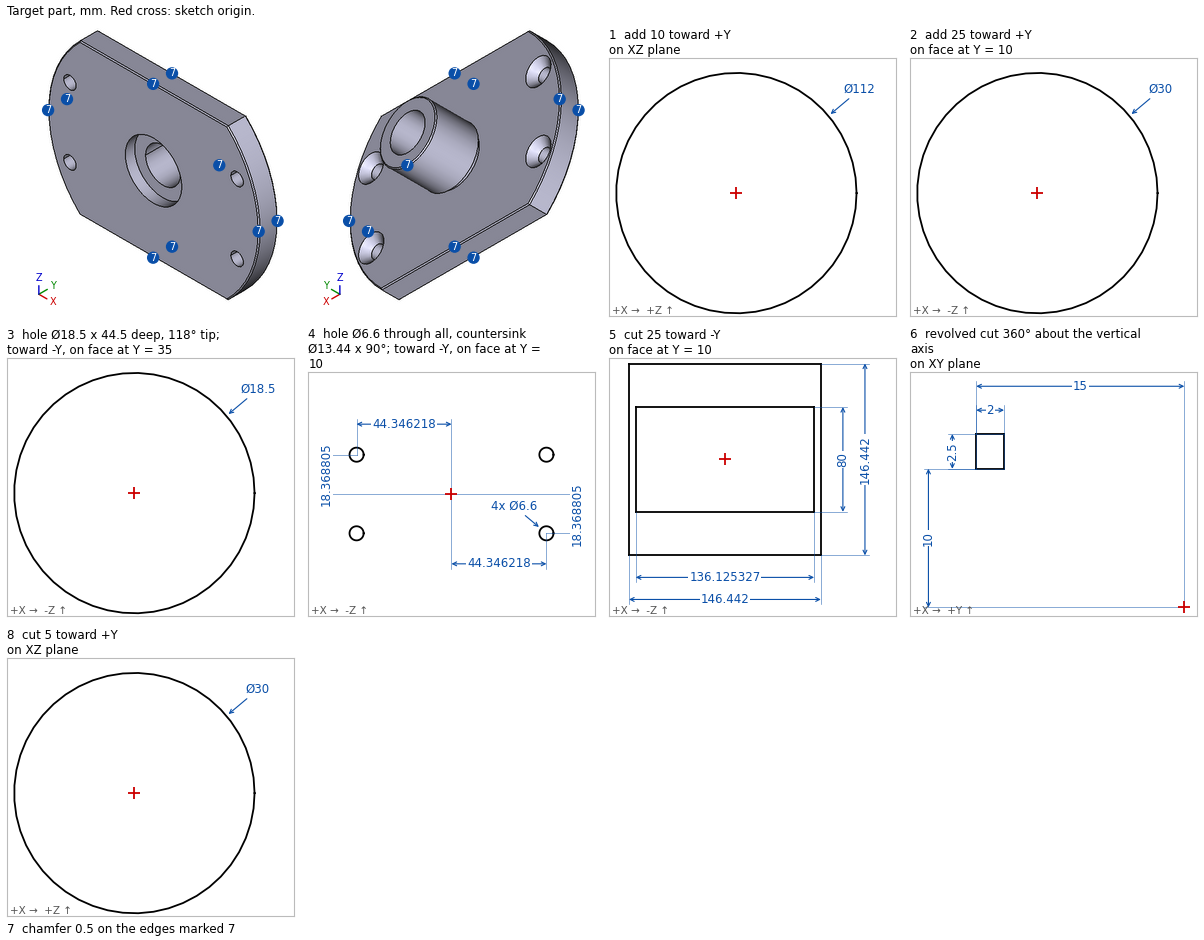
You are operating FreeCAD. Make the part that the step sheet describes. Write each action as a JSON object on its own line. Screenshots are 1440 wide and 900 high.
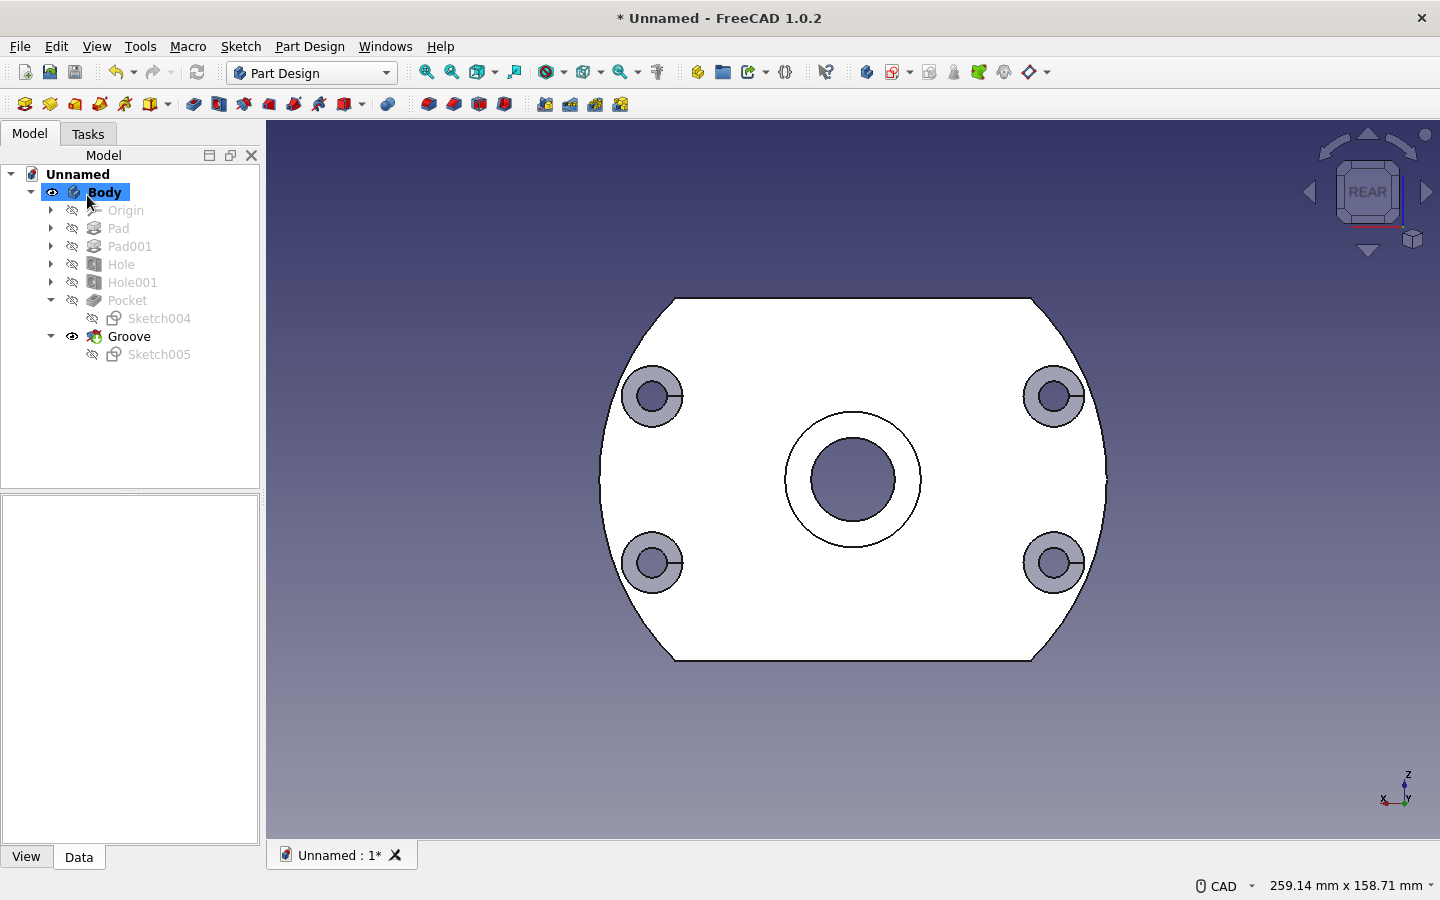
{"action": "left_click", "coordinate": [638, 613]}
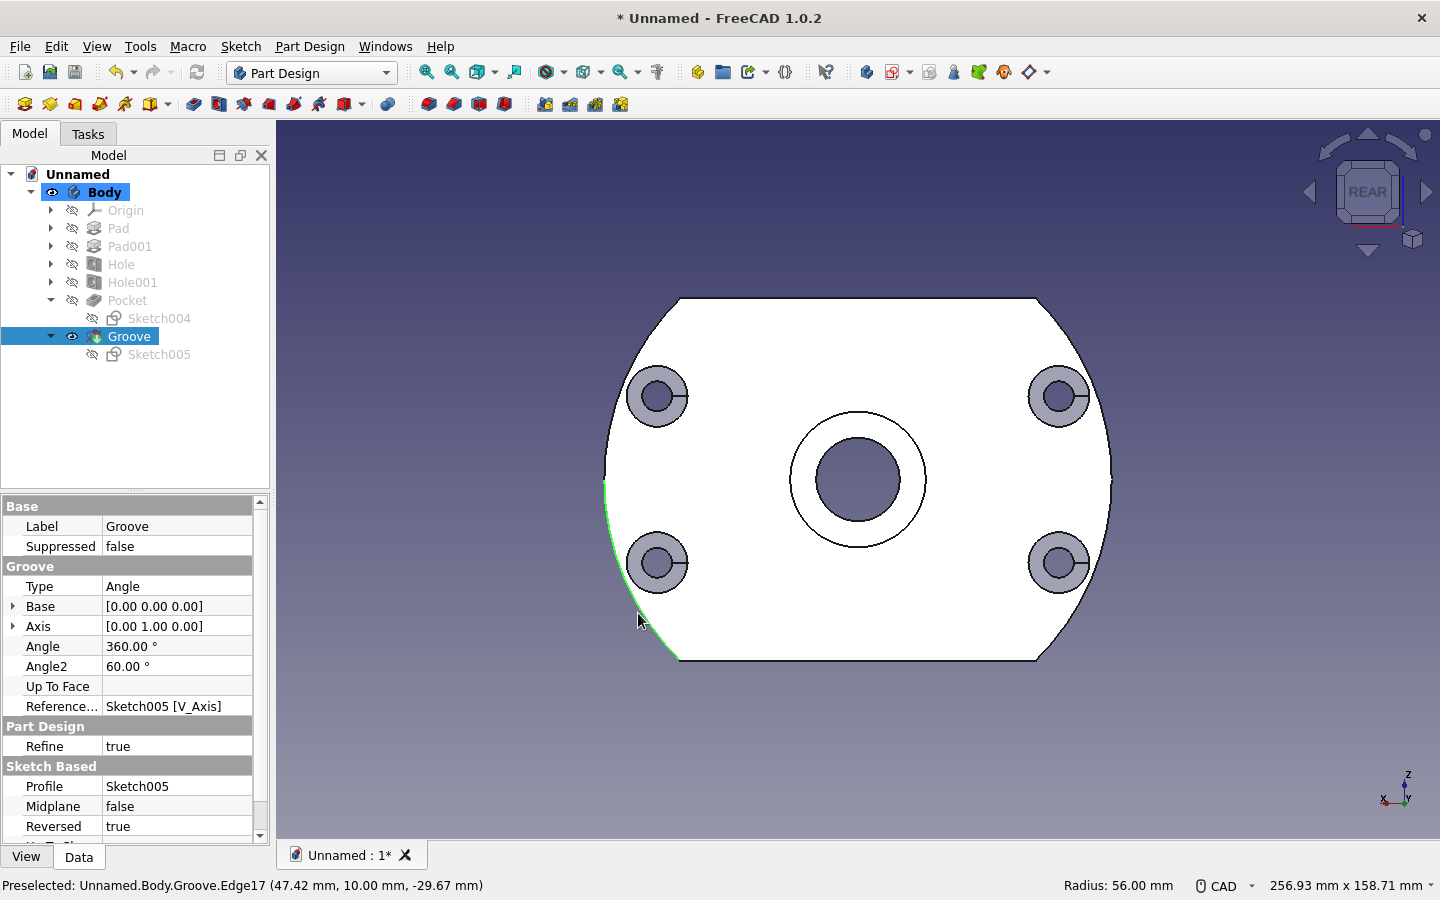
{"action": "left_click", "coordinate": [1112, 479], "text": "ctrl"}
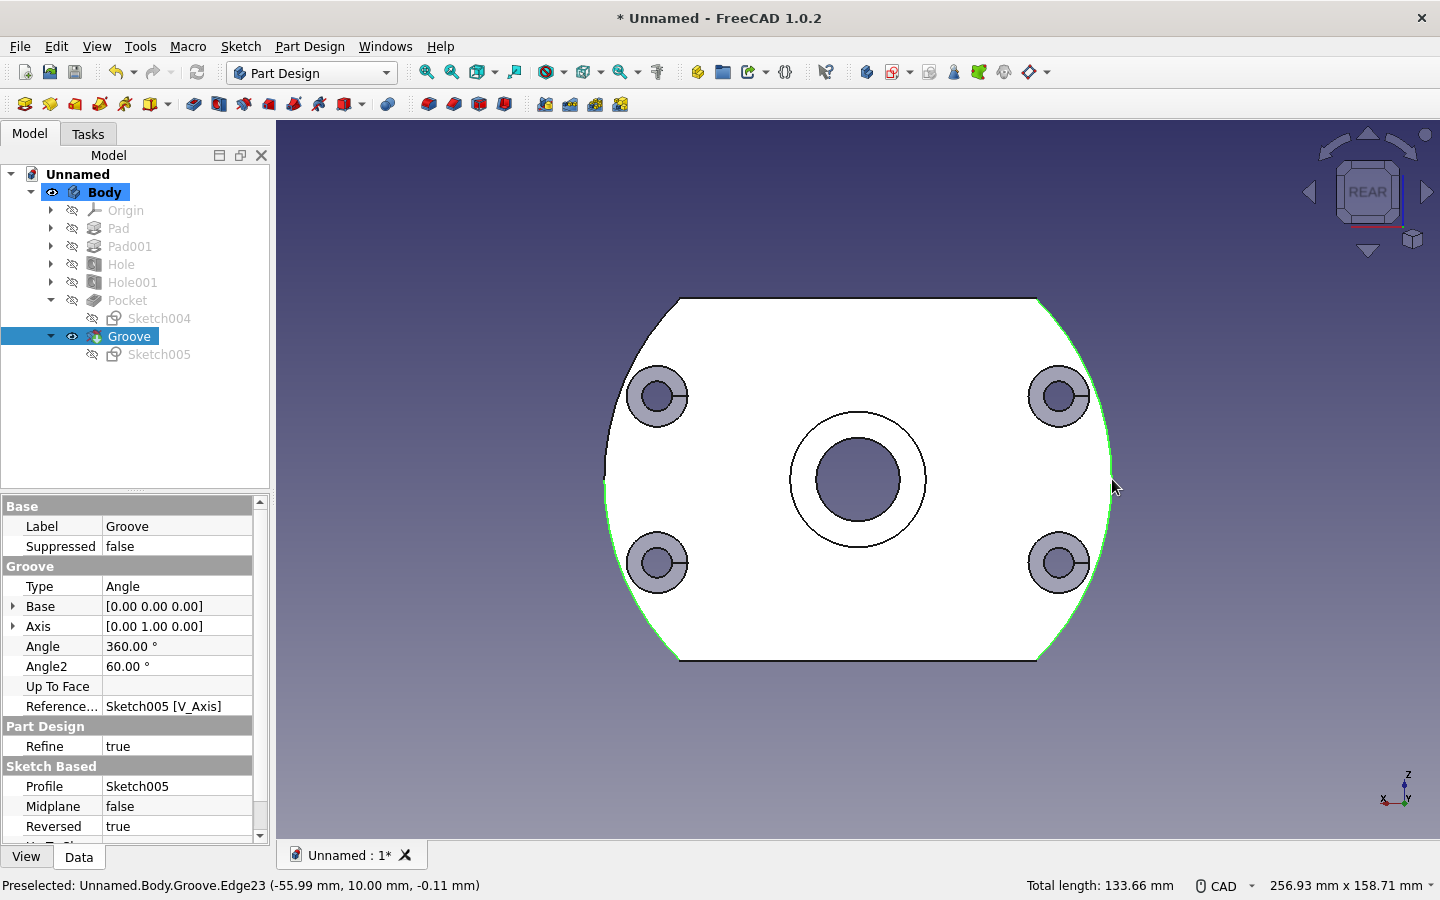
{"action": "left_click", "coordinate": [858, 660], "text": "ctrl"}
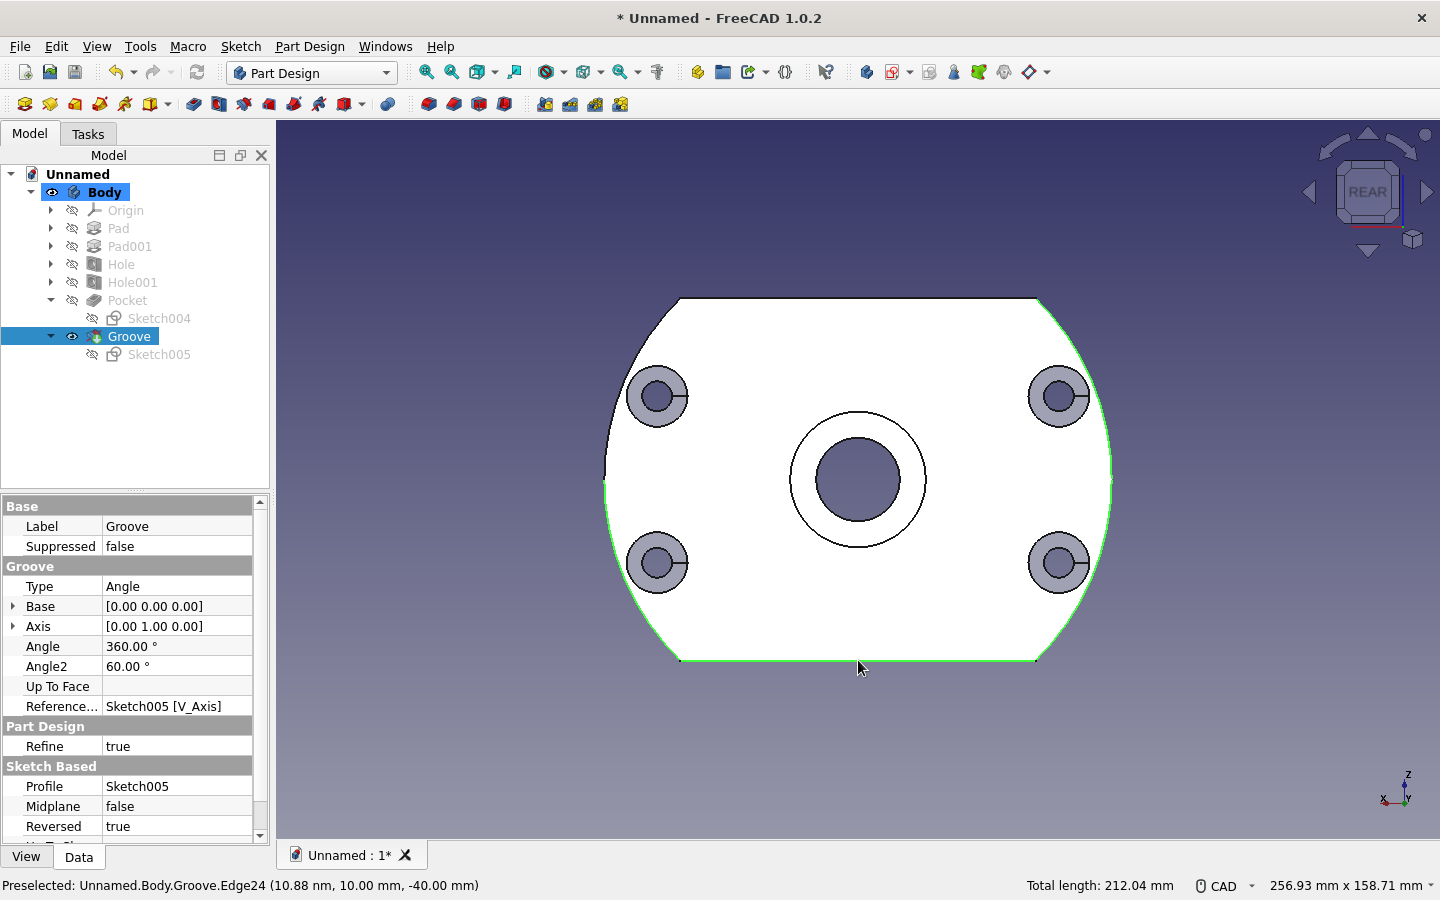
{"action": "left_click", "coordinate": [926, 478], "text": "ctrl"}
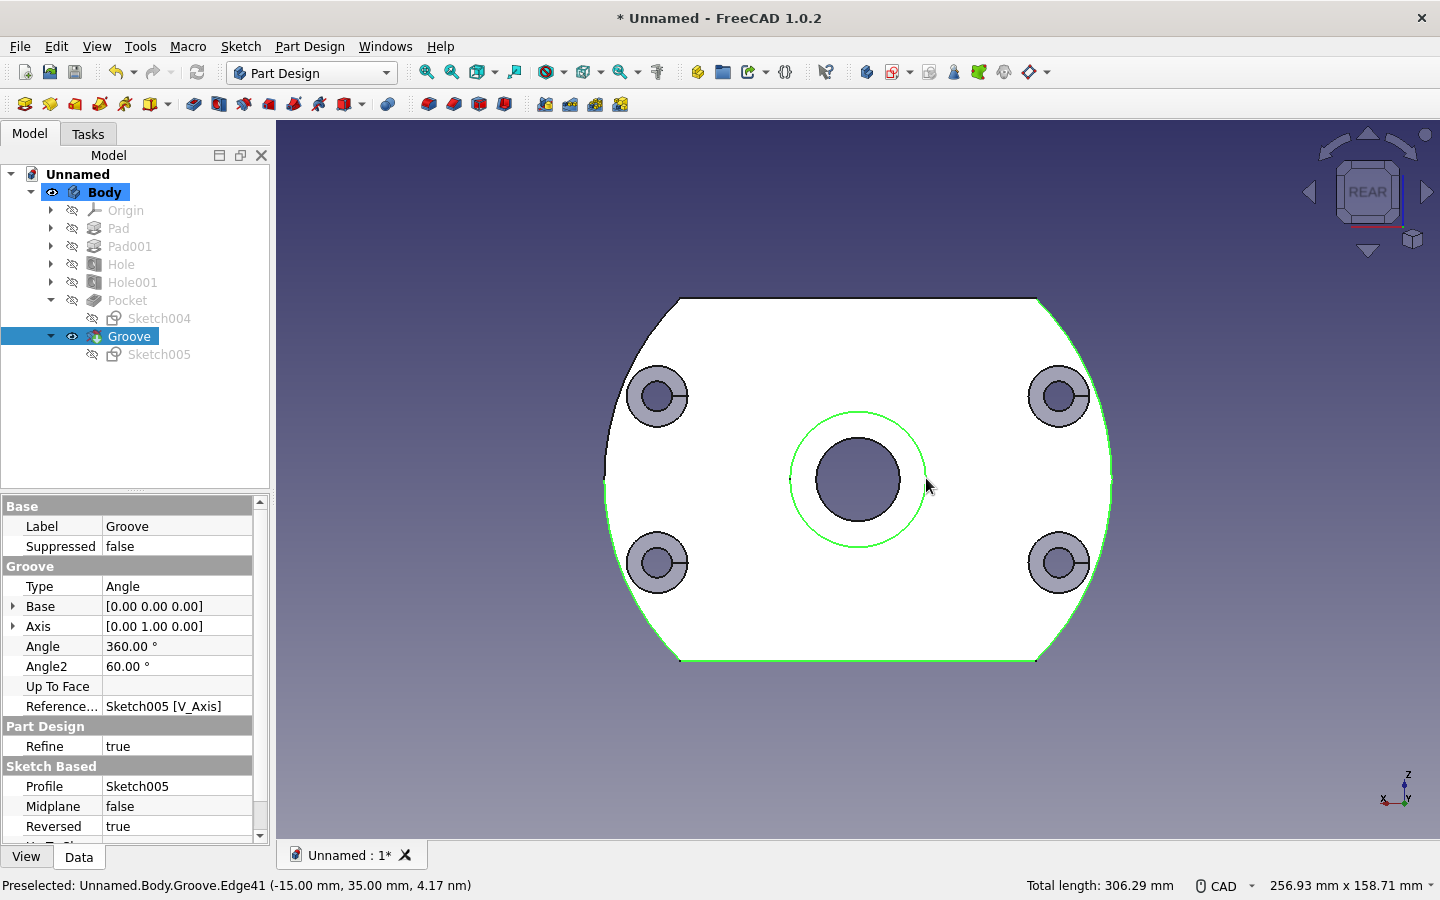
{"action": "key", "text": "0"}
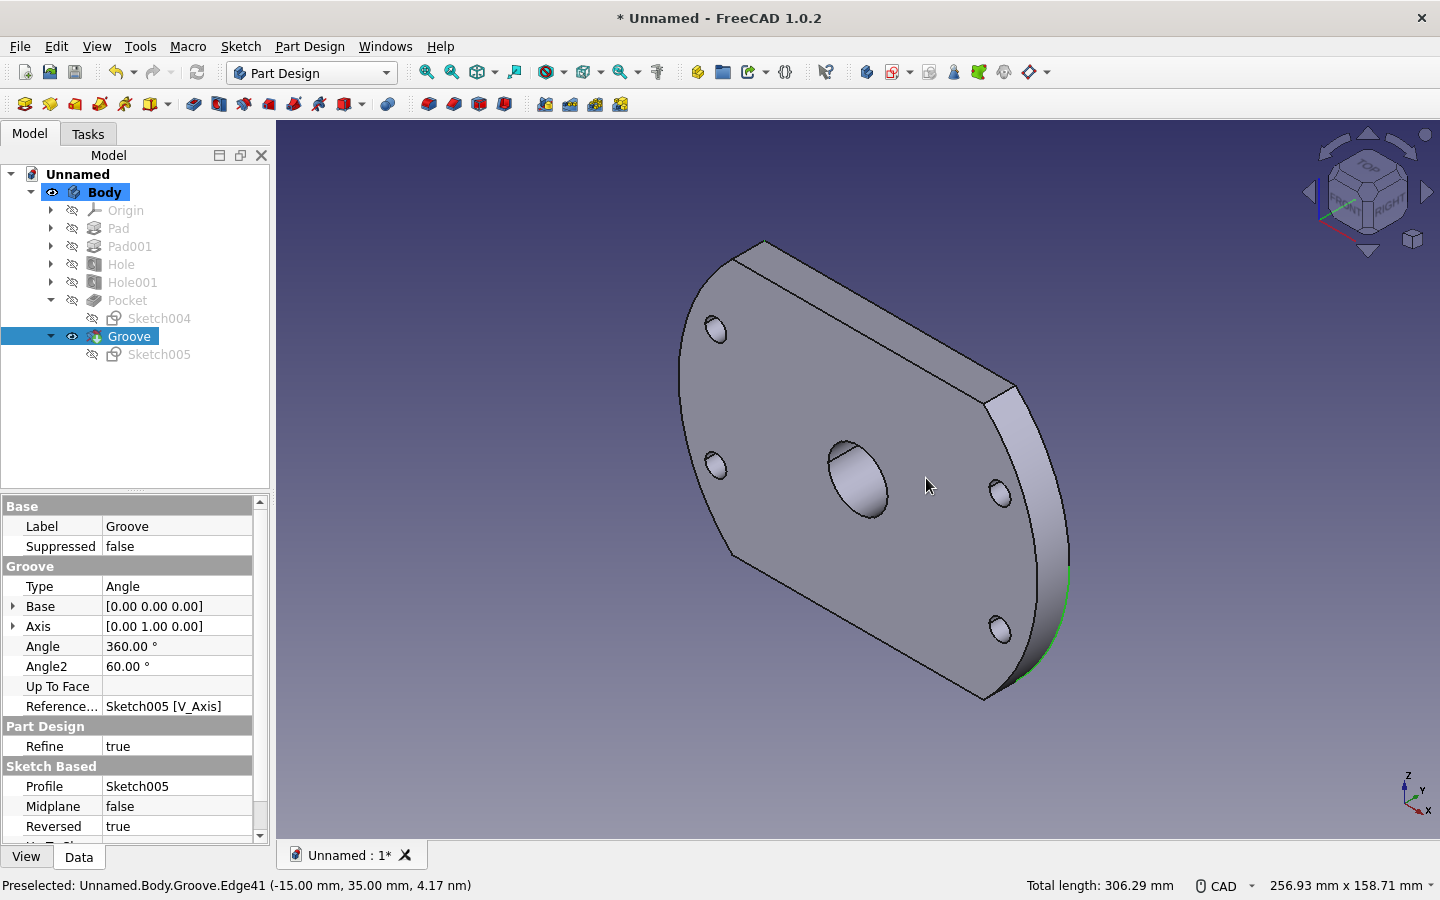
{"action": "left_click", "coordinate": [1023, 494], "text": "ctrl"}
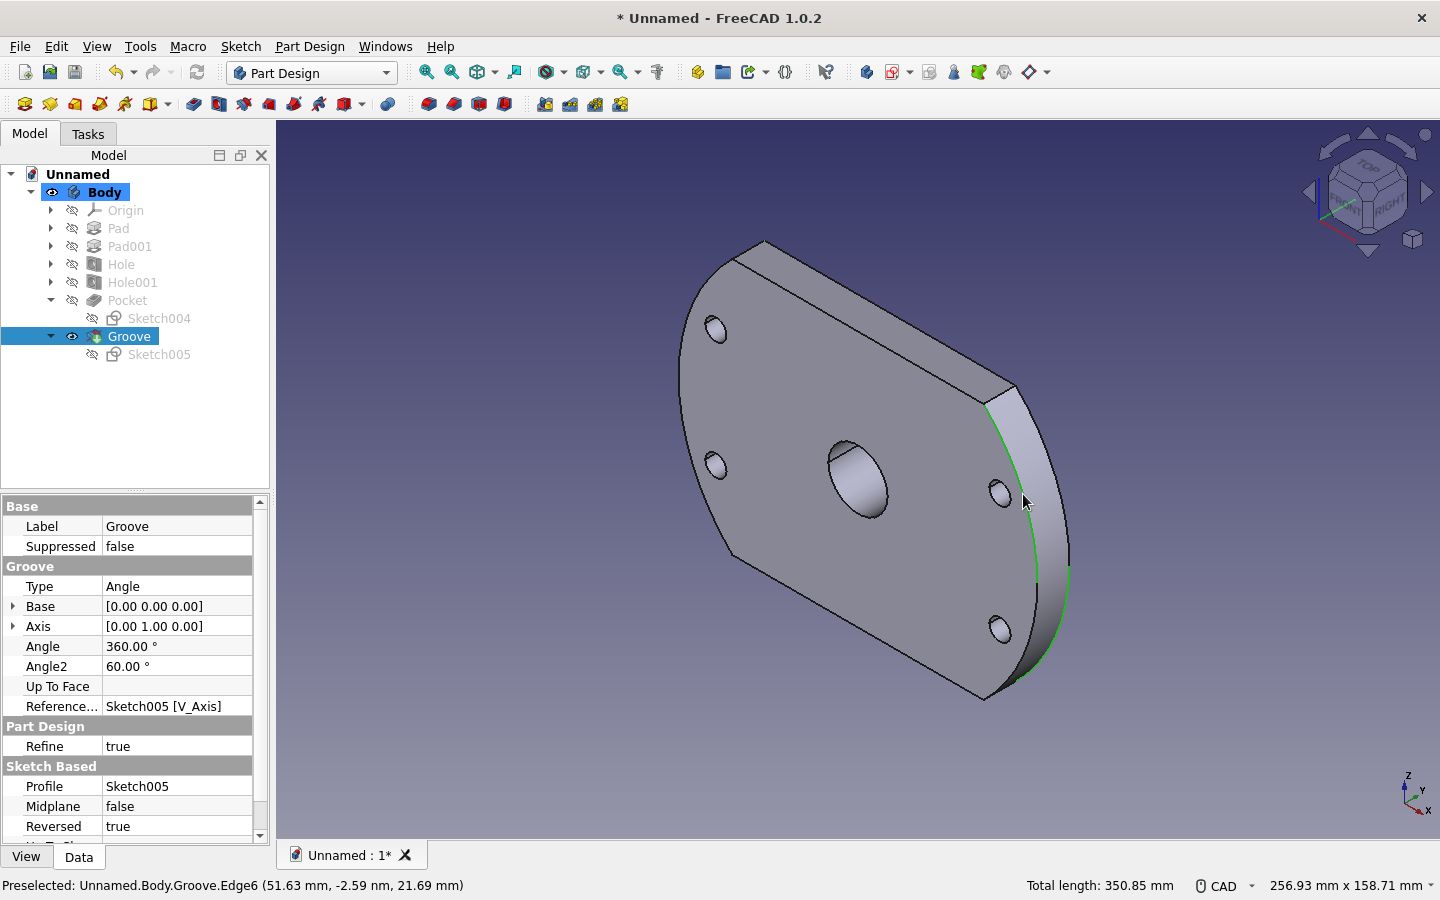
{"action": "left_click", "coordinate": [858, 331], "text": "ctrl"}